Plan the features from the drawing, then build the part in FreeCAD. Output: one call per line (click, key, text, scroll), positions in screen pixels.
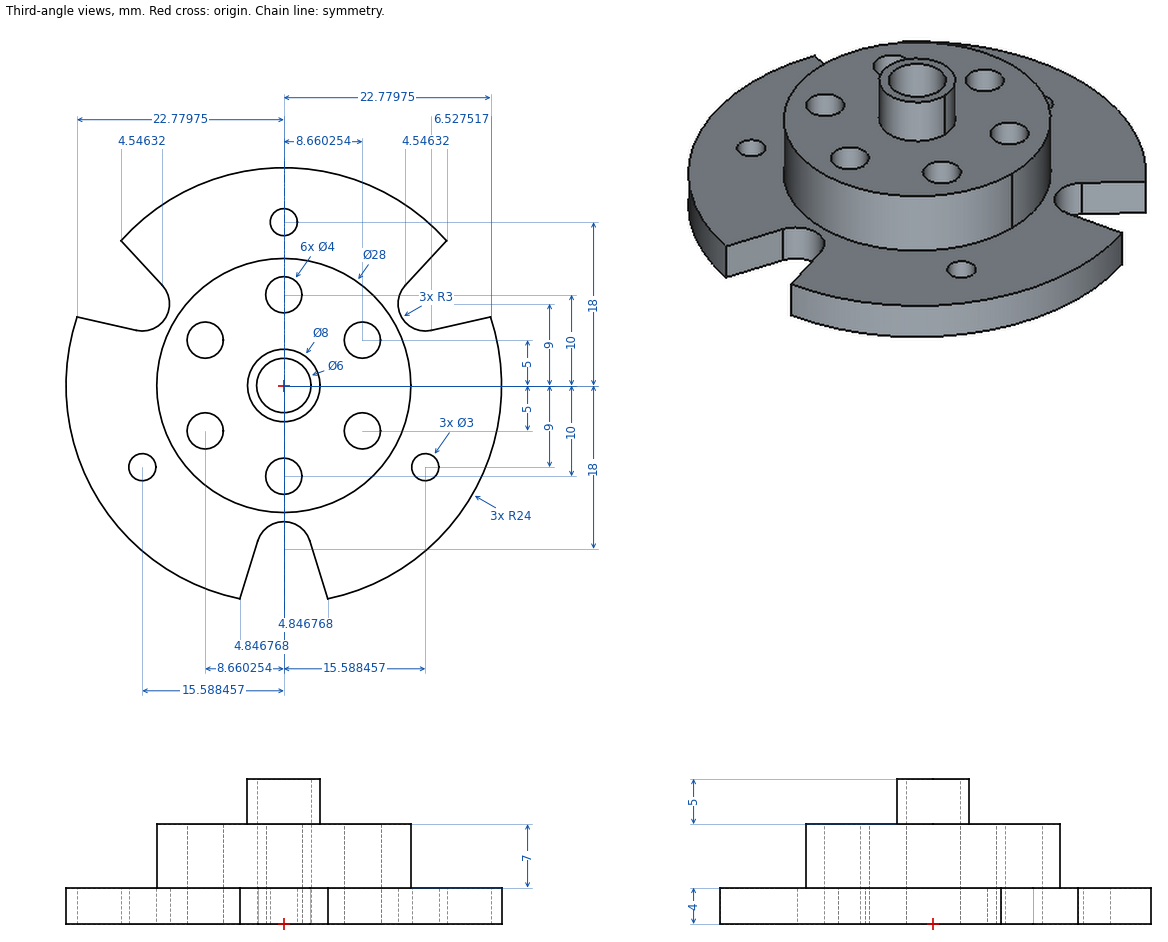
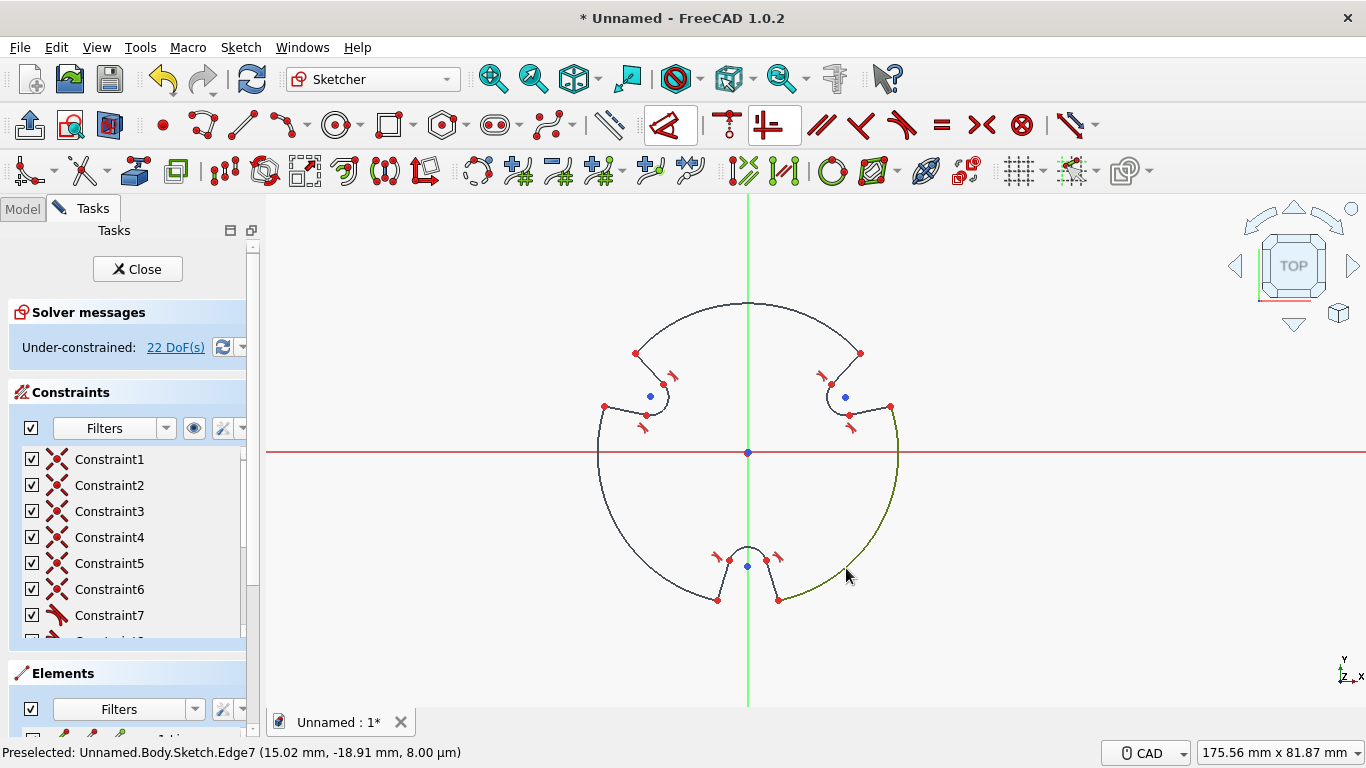
click(600, 481)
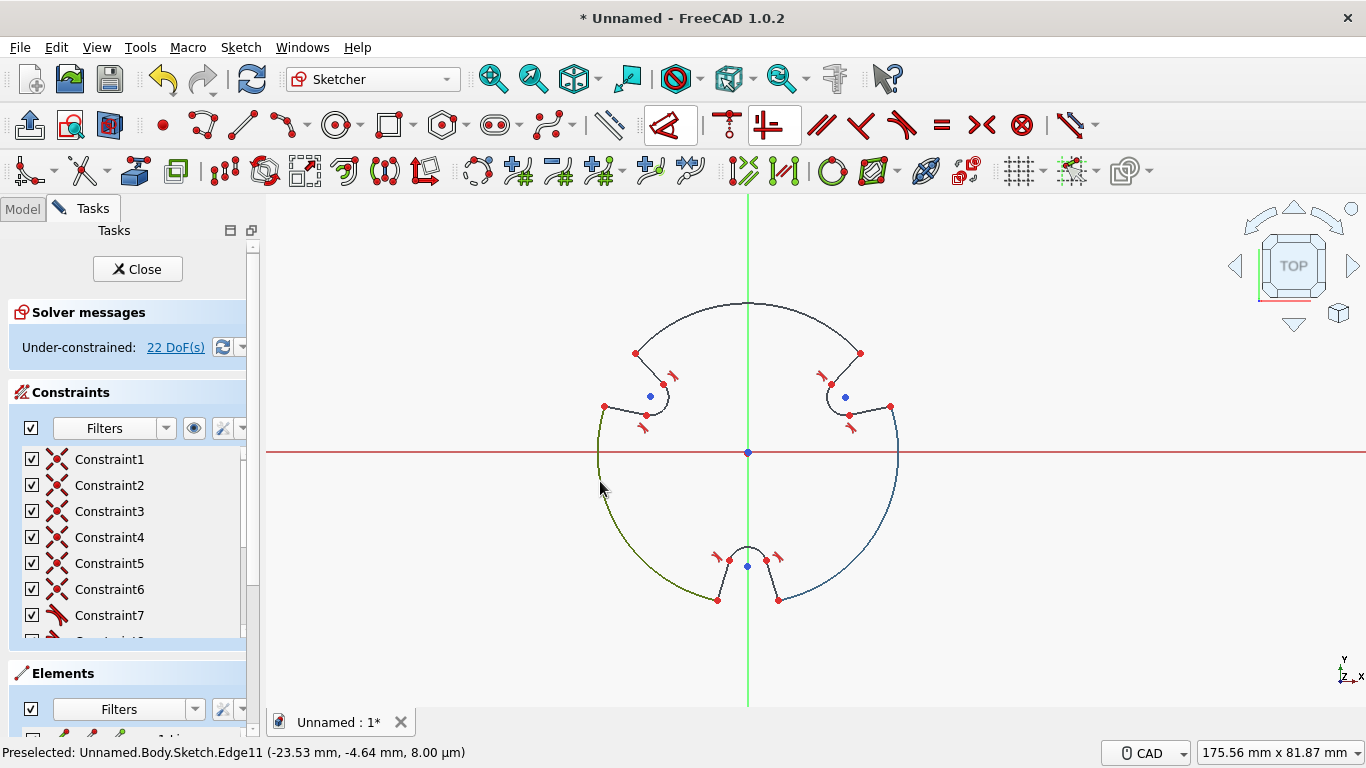
click(728, 126)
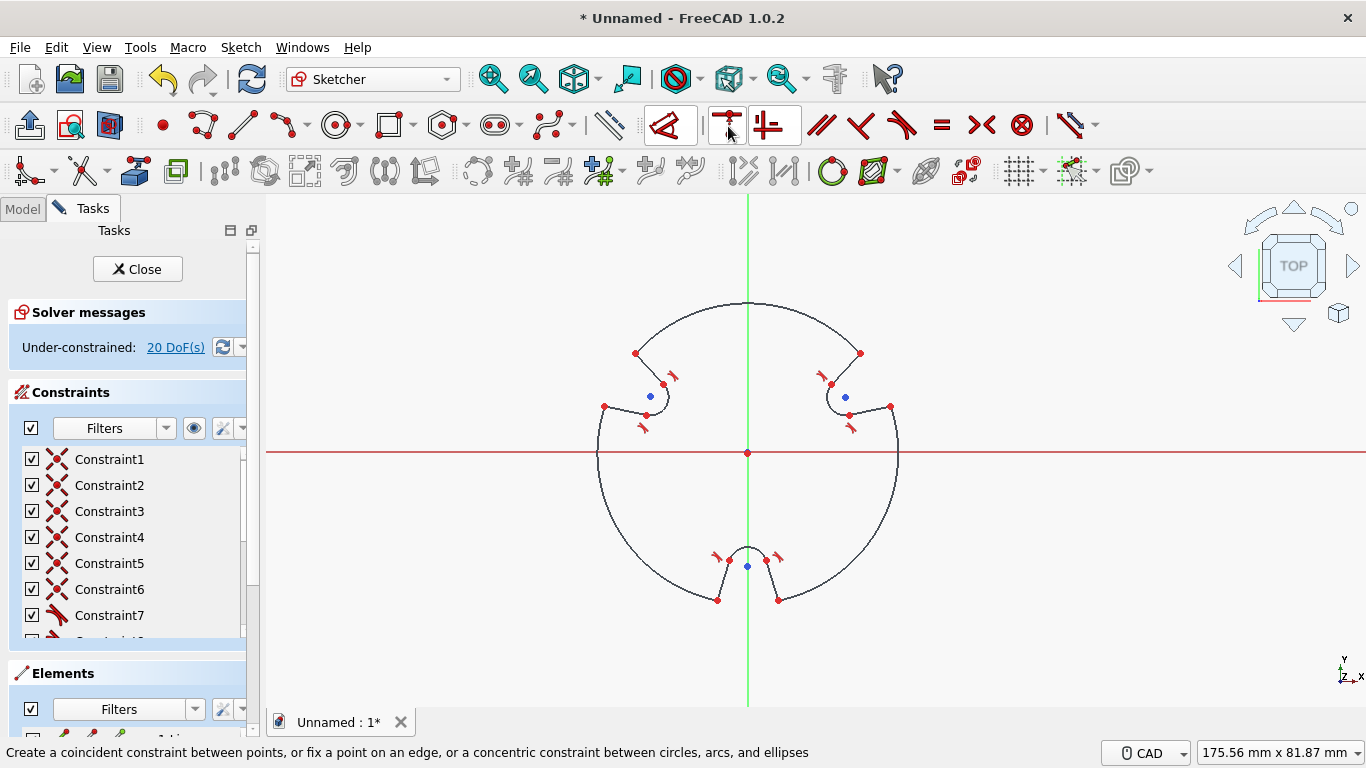
scroll(748, 453, up, 4)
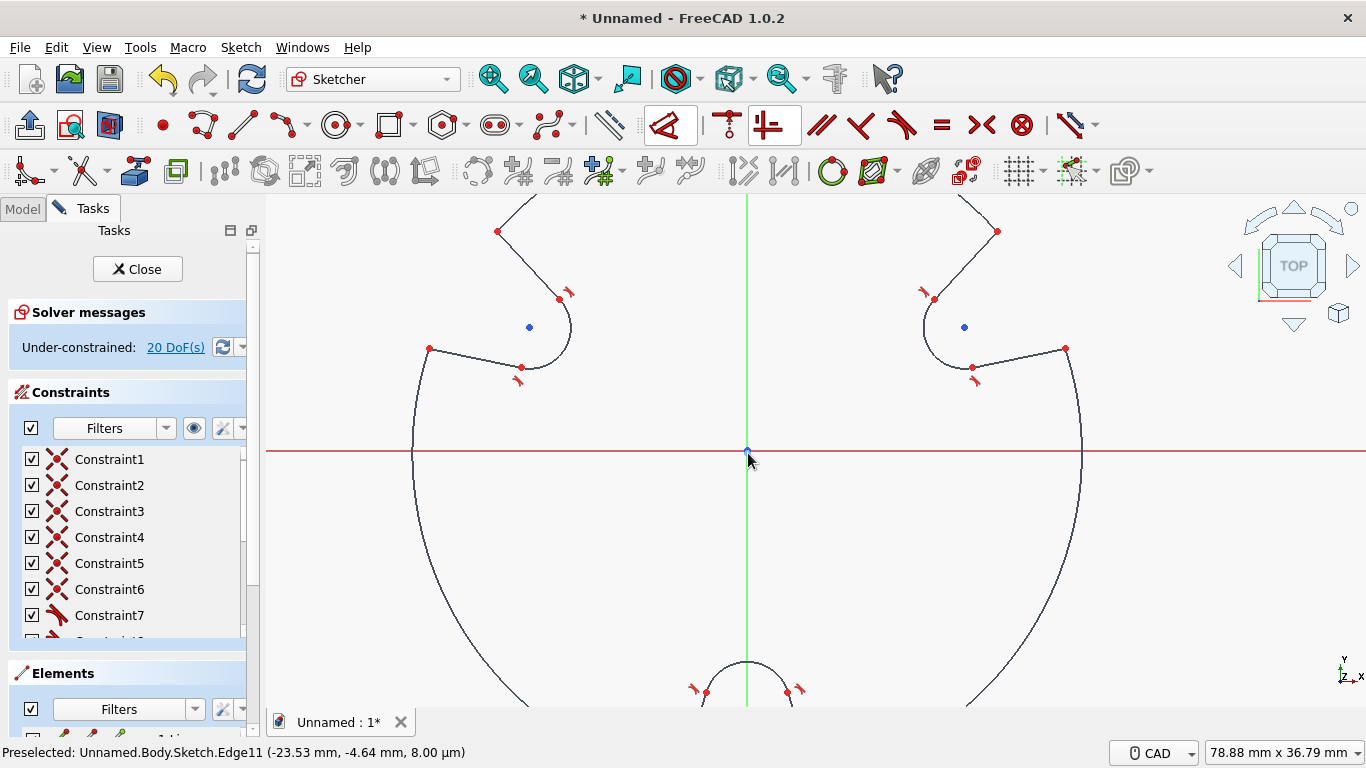
drag(737, 441, 757, 463)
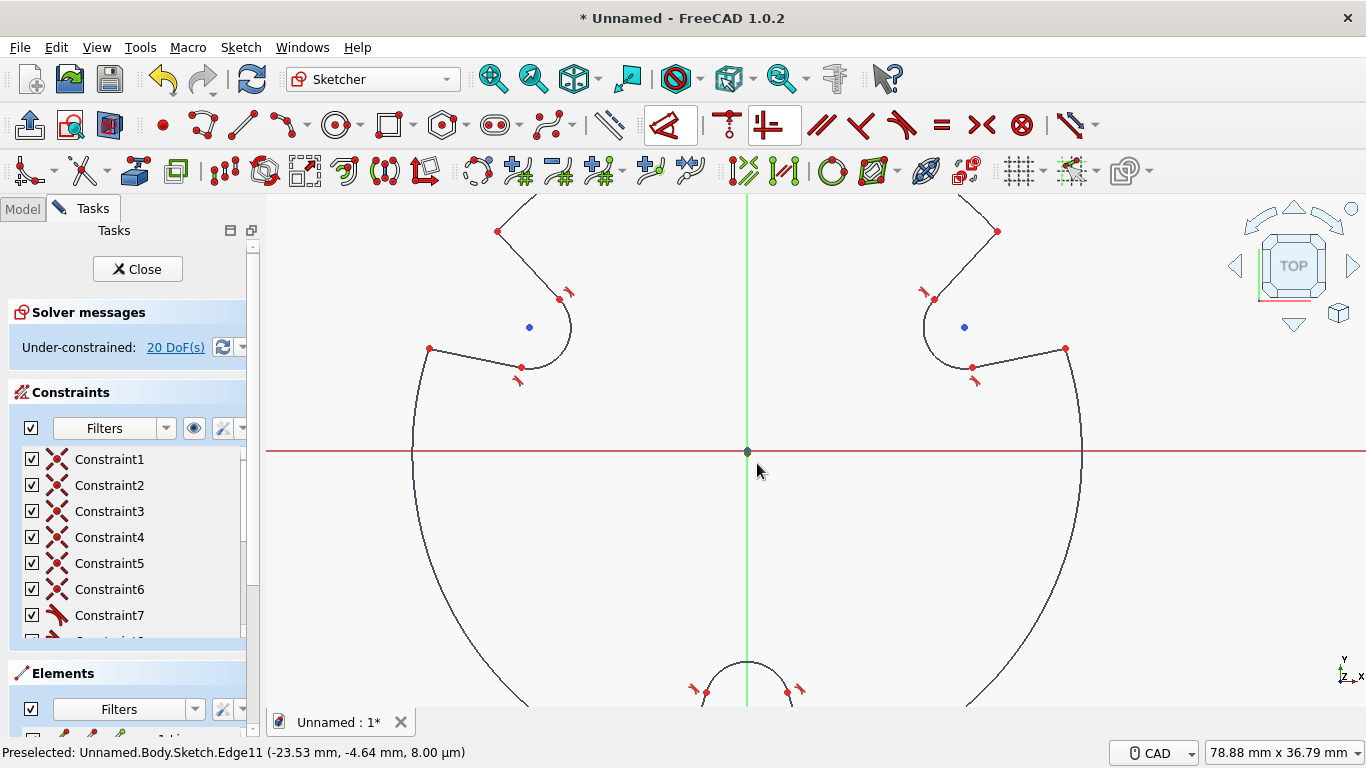
key(c)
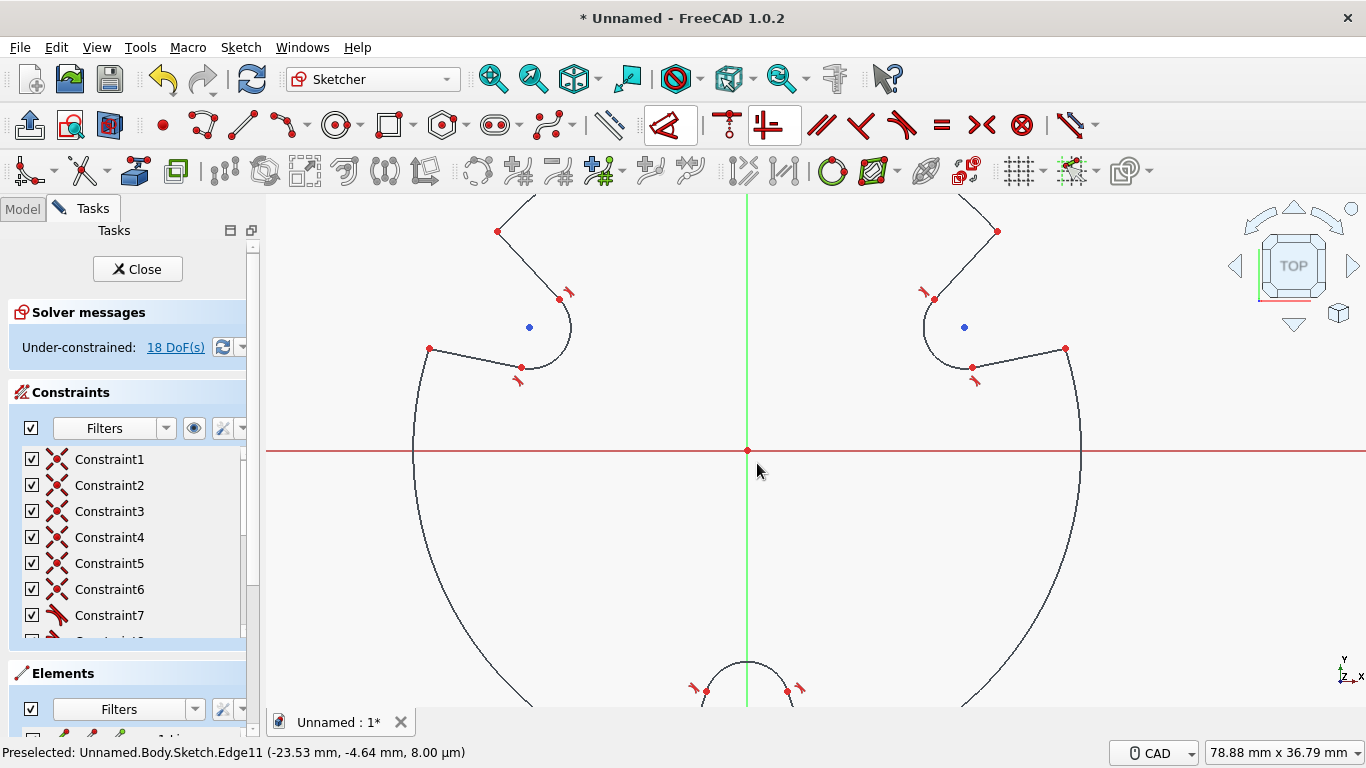
click(1075, 515)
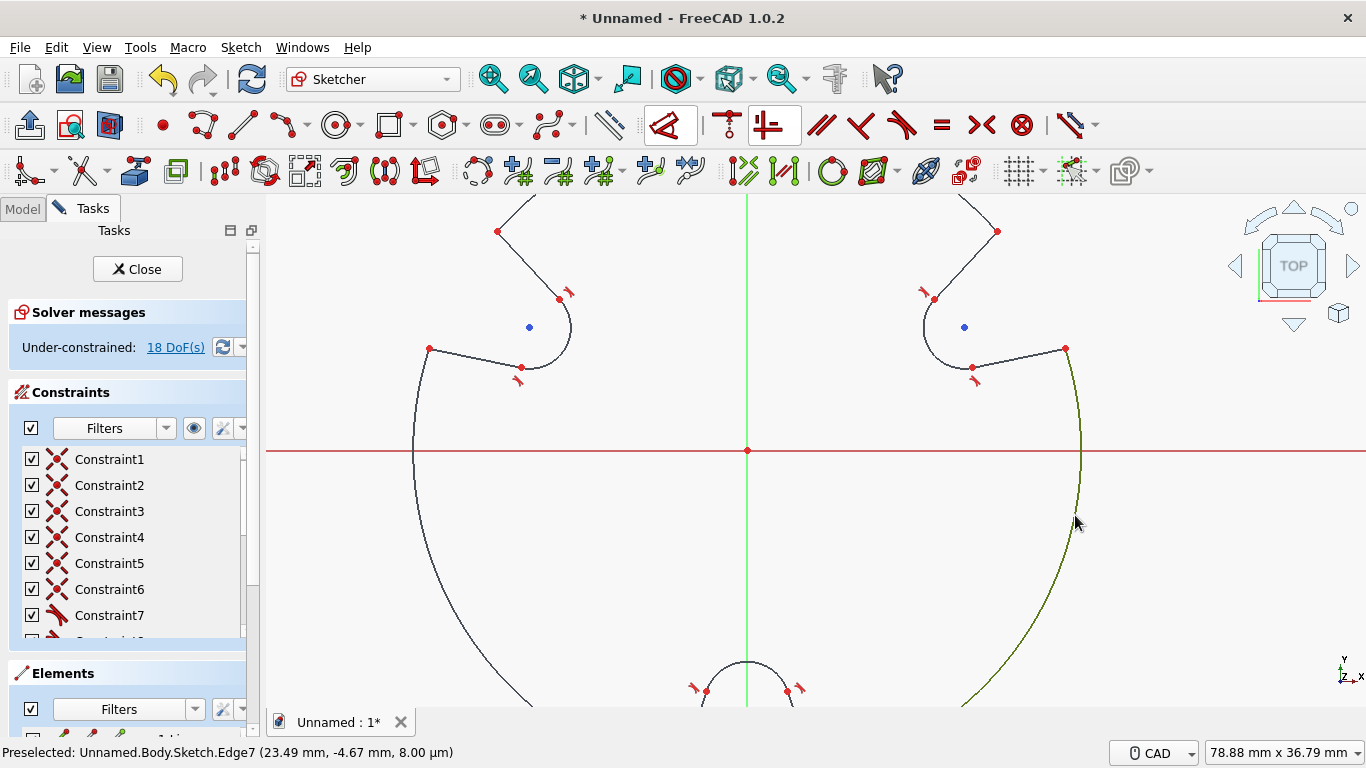
scroll(748, 453, down, 4)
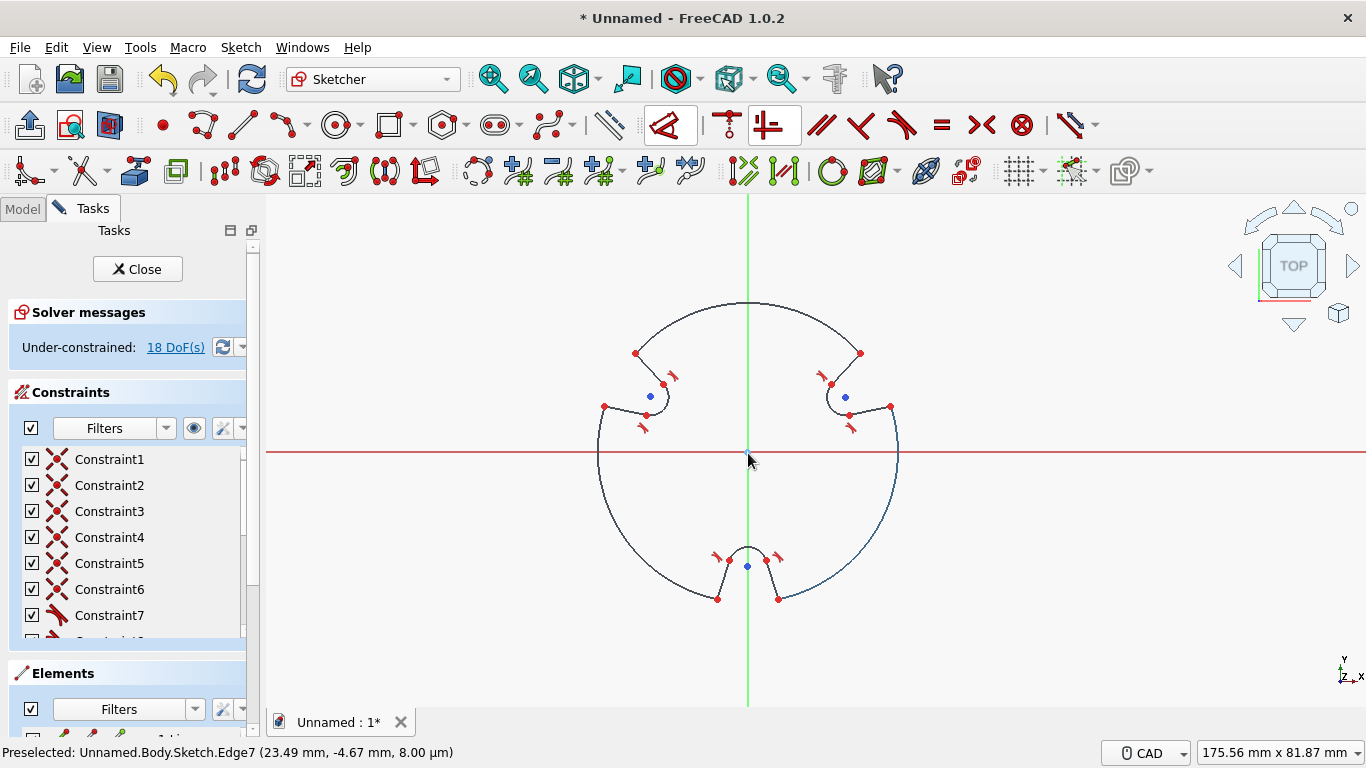
click(798, 312)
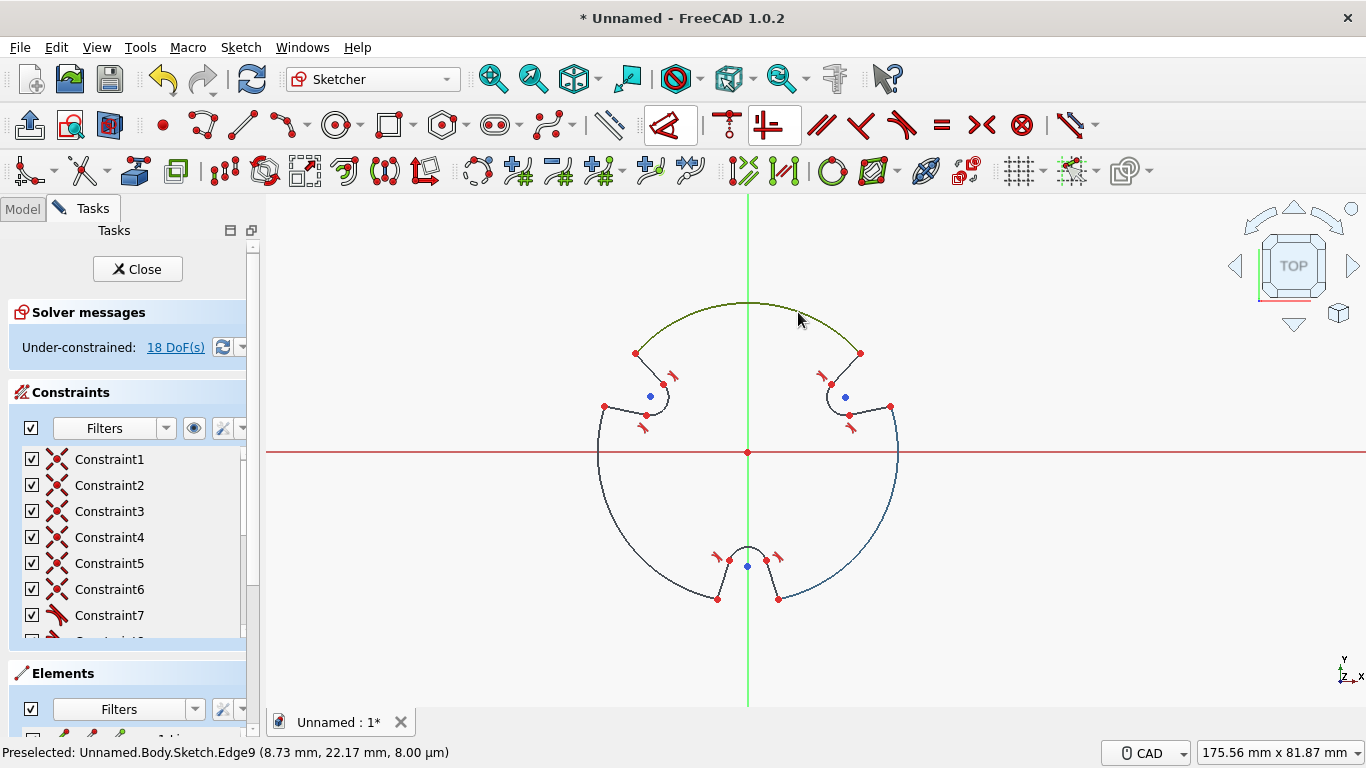
click(601, 481)